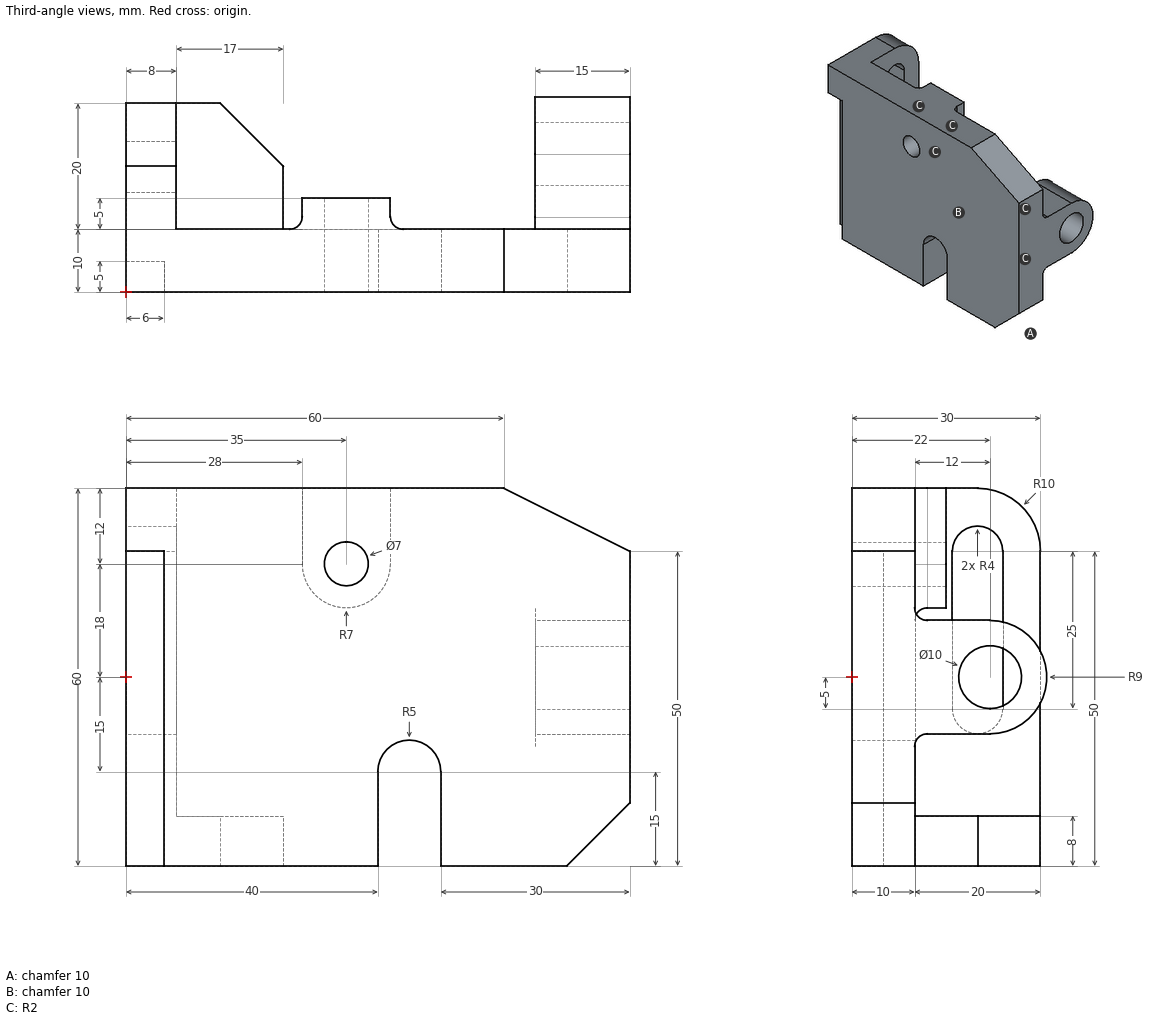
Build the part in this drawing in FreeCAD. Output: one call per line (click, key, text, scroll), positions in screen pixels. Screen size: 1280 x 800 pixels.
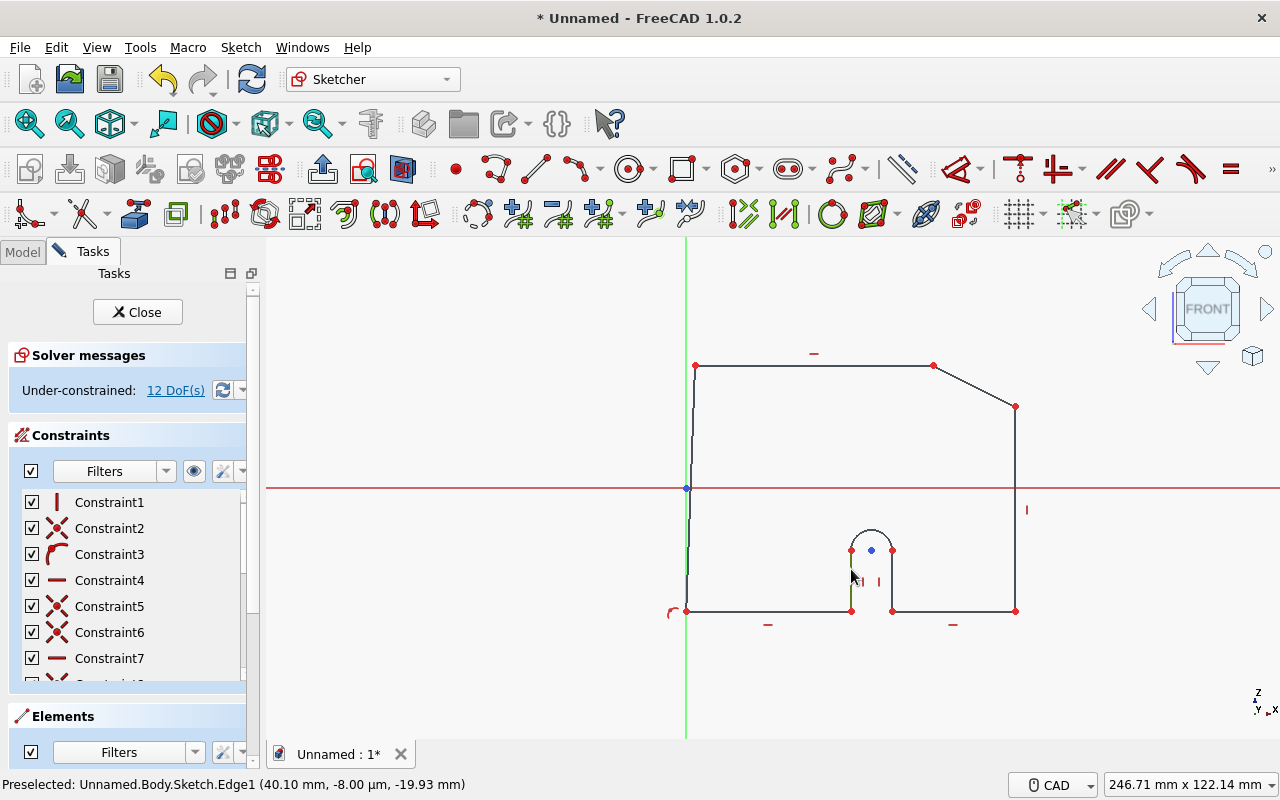
click(884, 534)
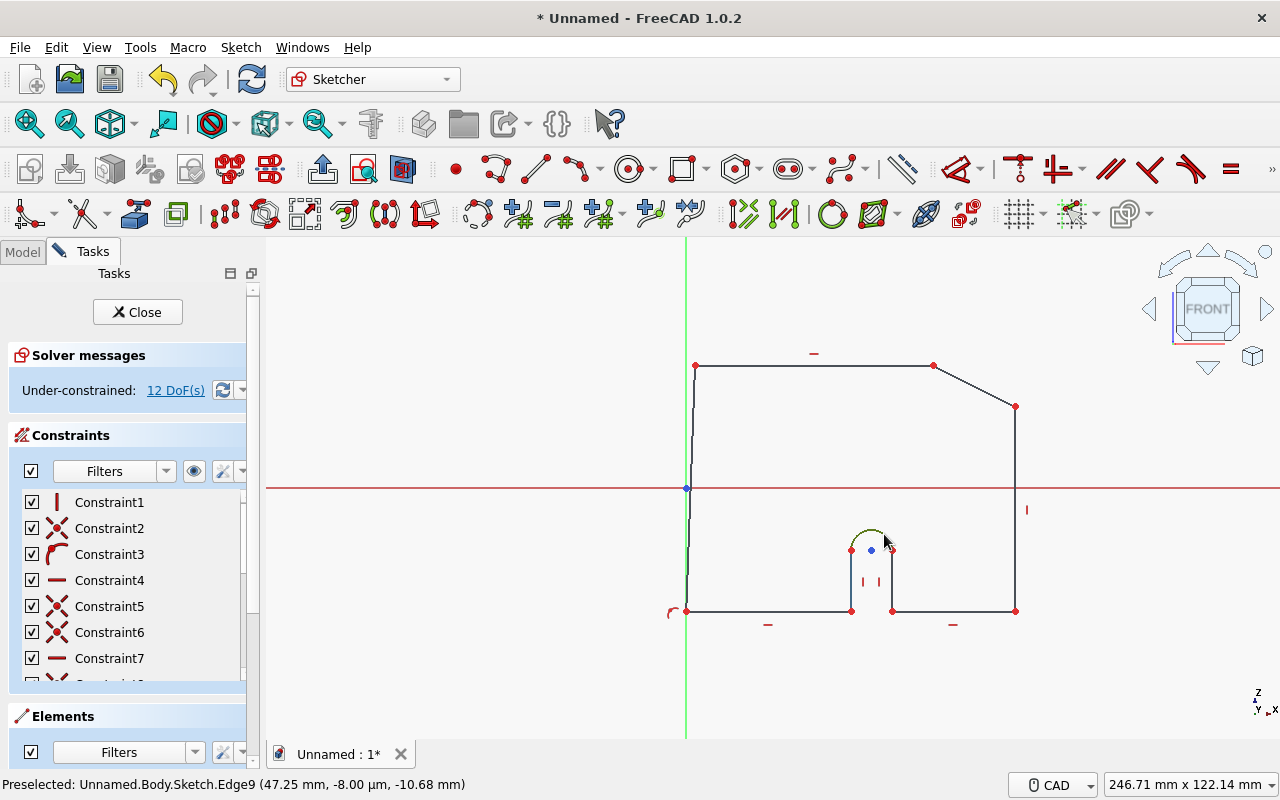
click(1192, 170)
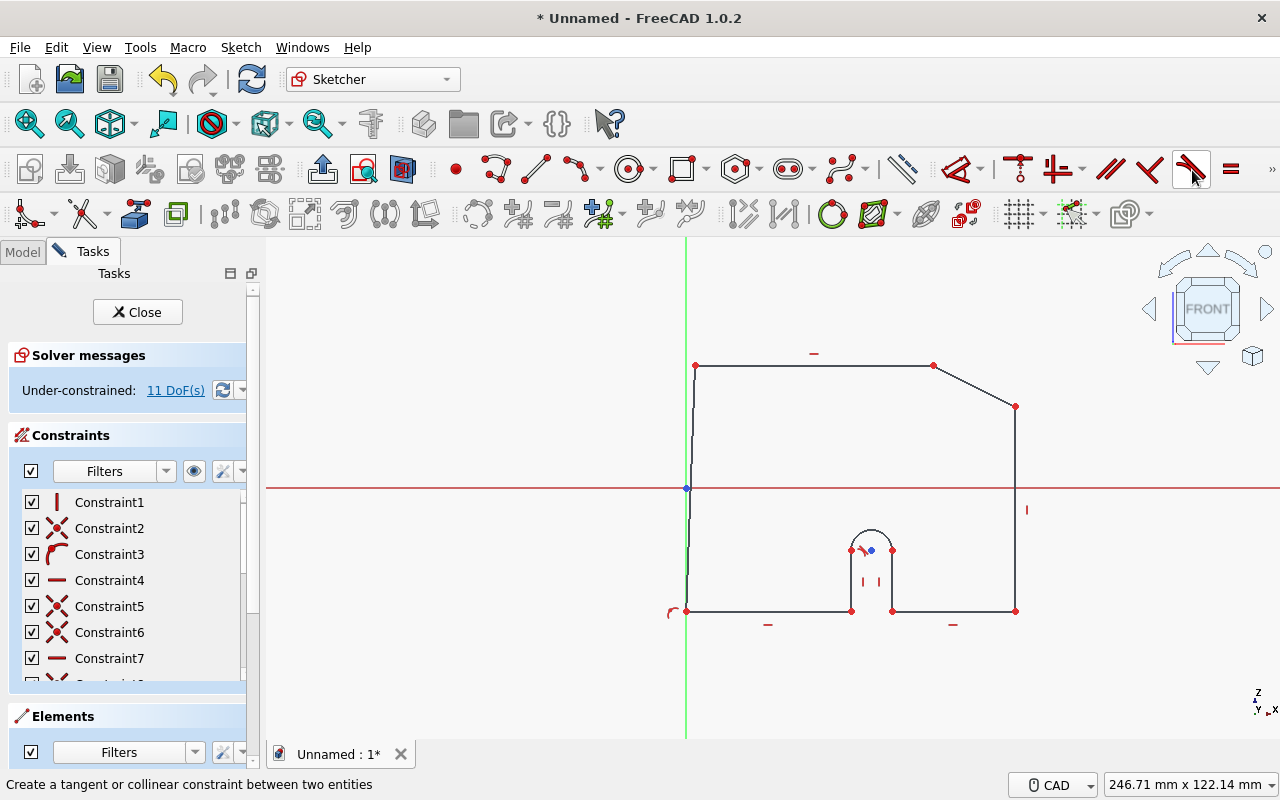
click(892, 594)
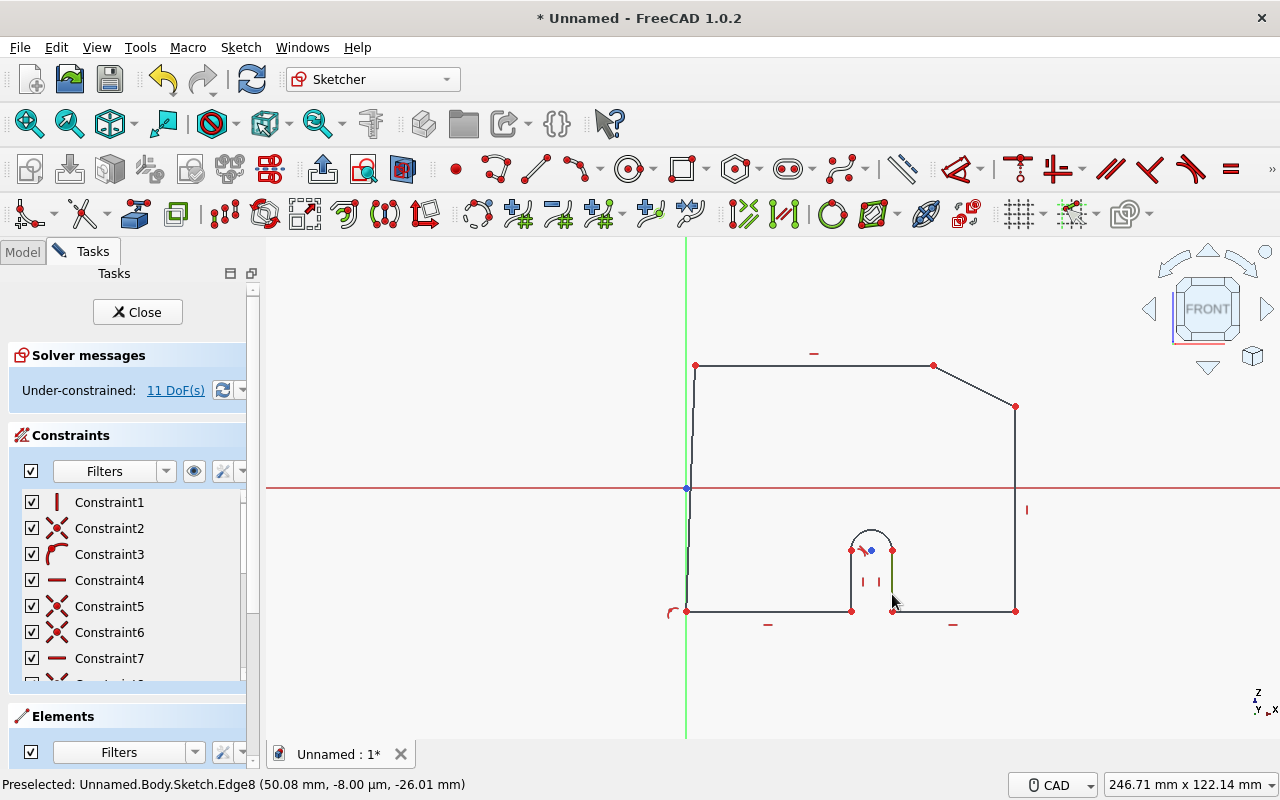
click(884, 534)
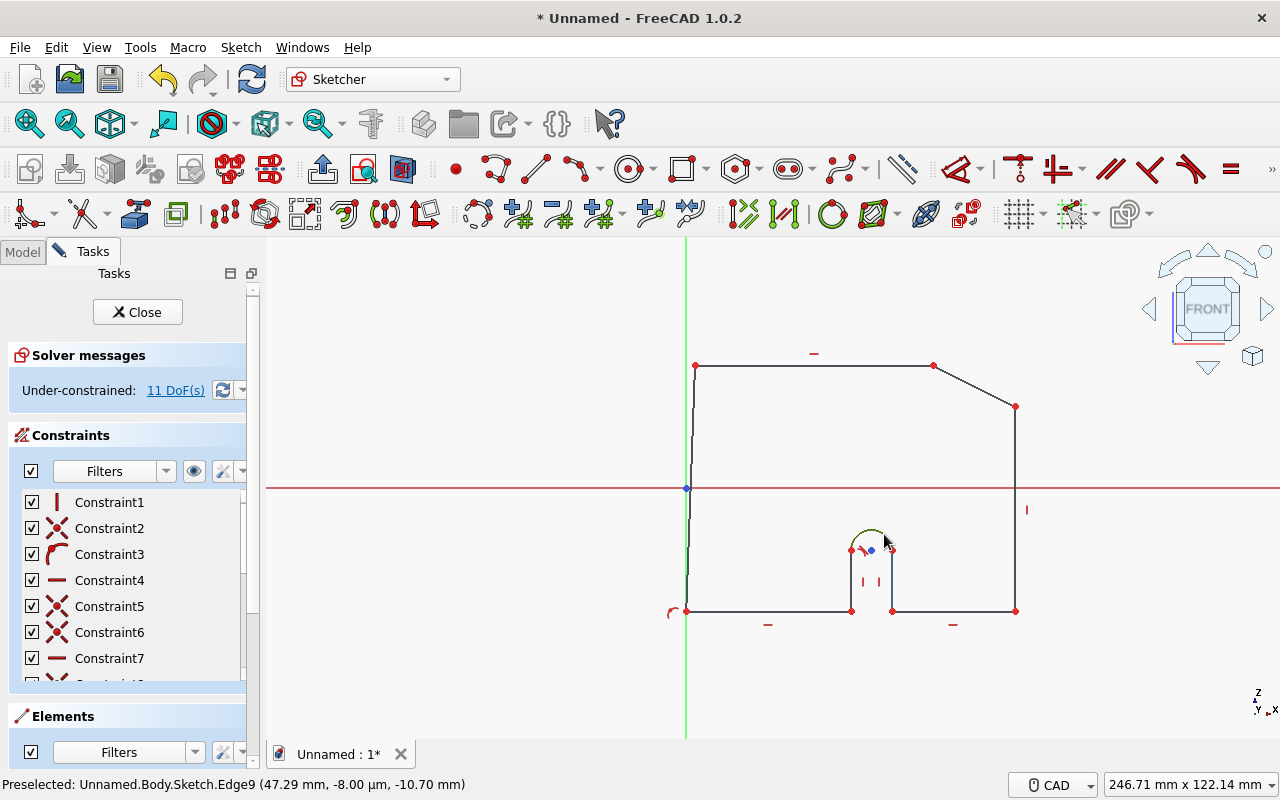
click(1192, 170)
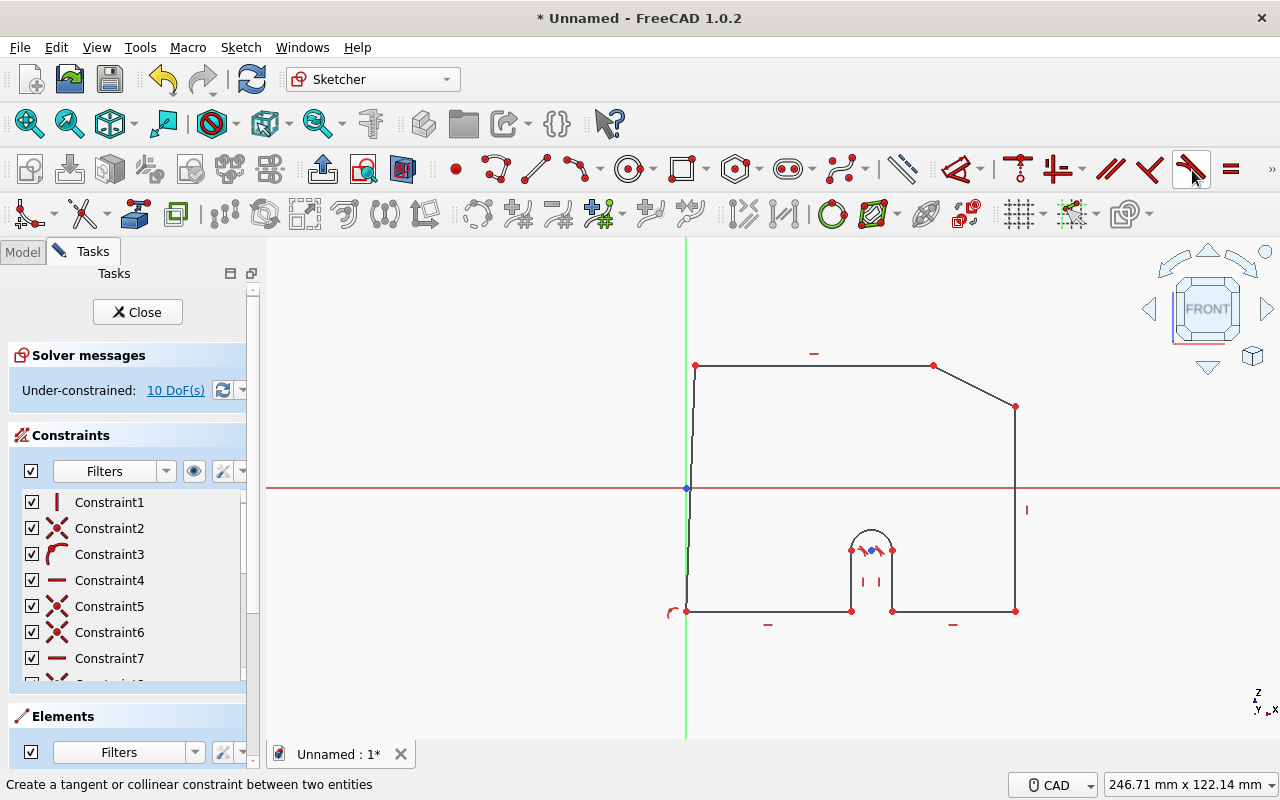
click(689, 538)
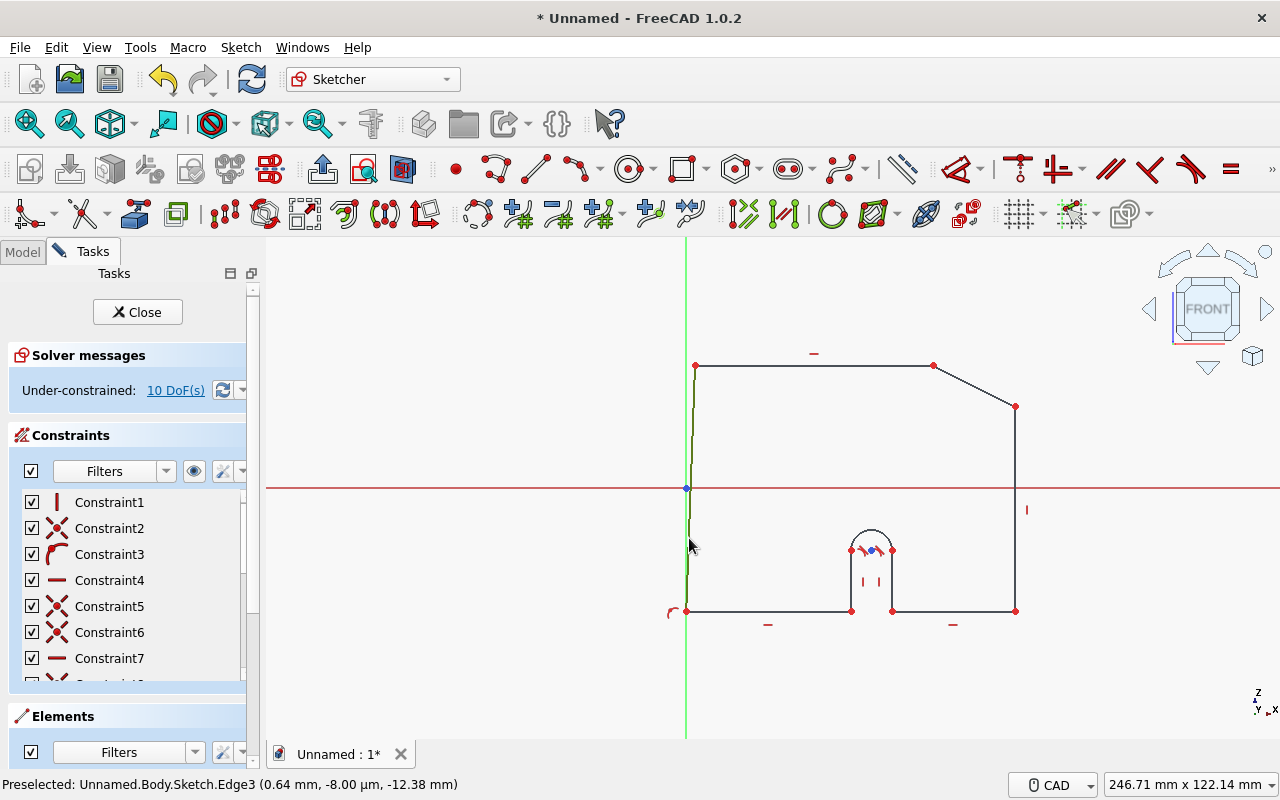
key(v)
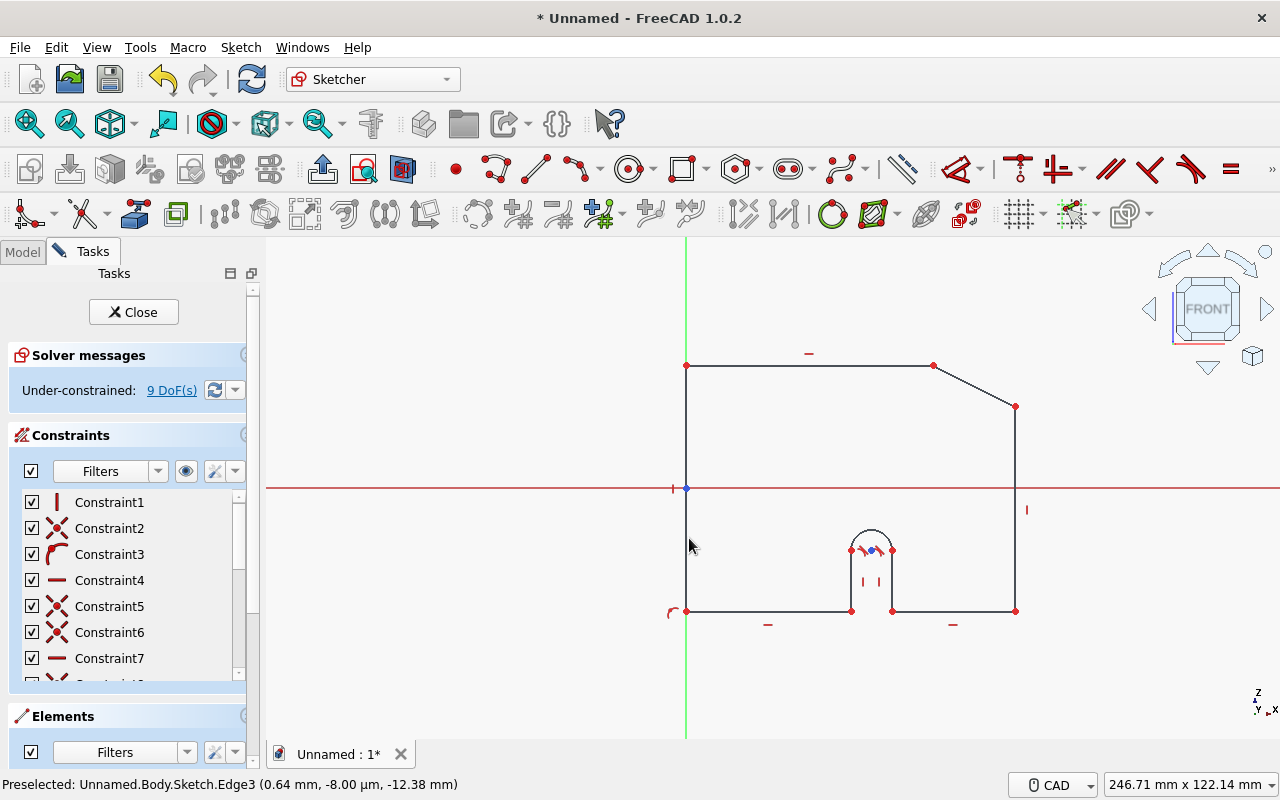
click(956, 170)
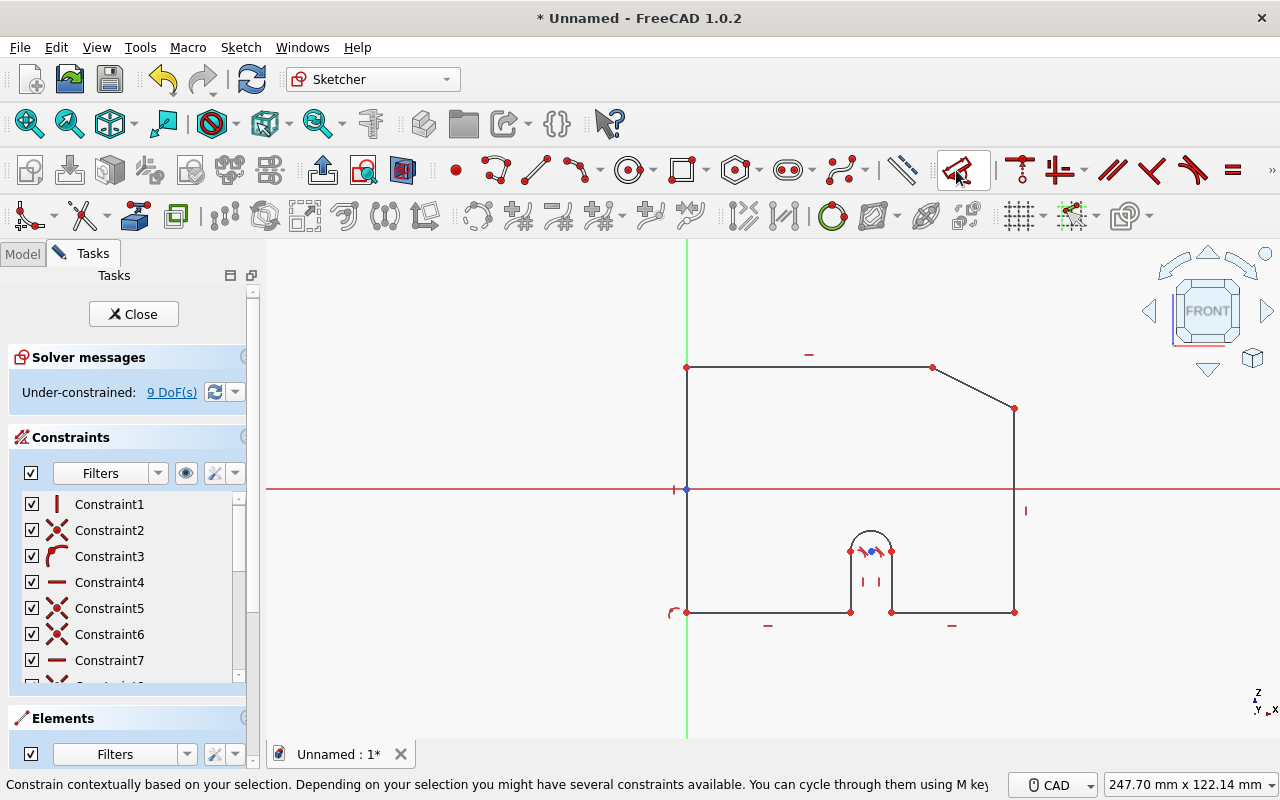
scroll(883, 535, up, 4)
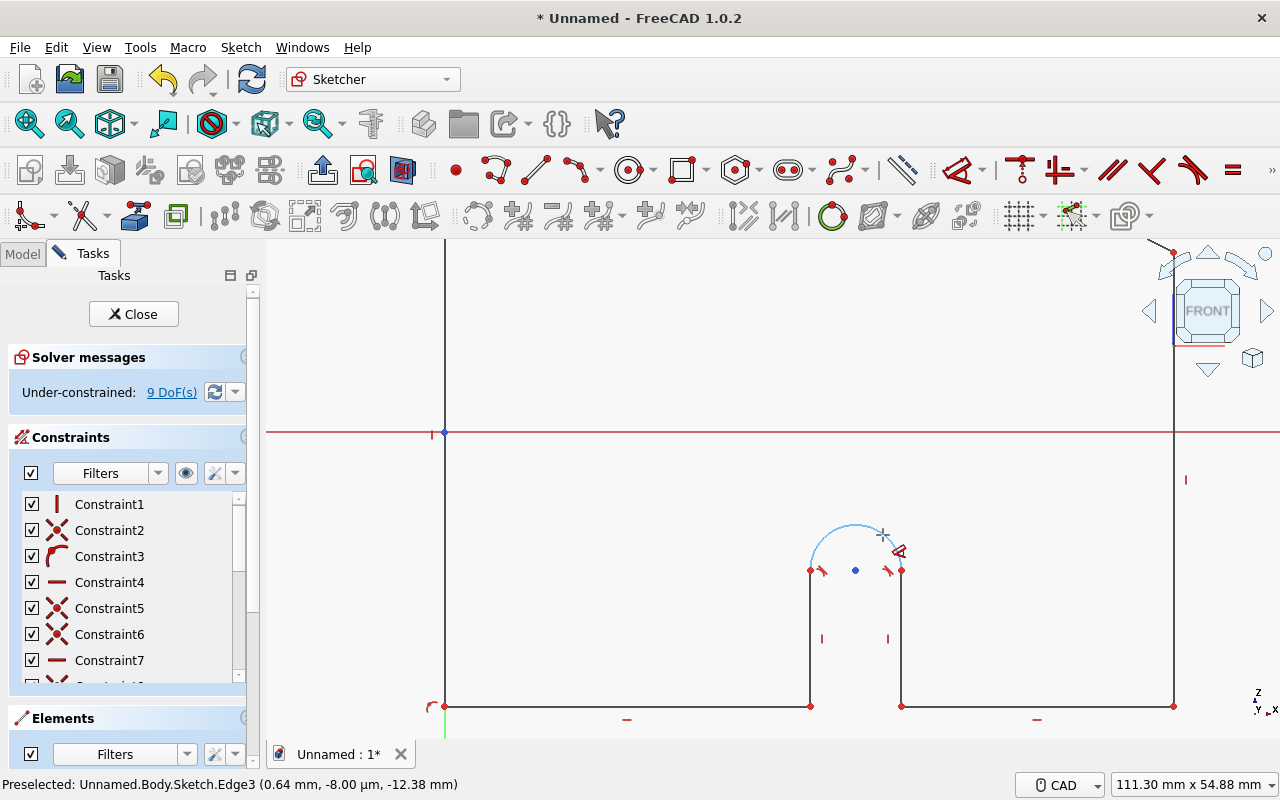
click(882, 534)
click(901, 508)